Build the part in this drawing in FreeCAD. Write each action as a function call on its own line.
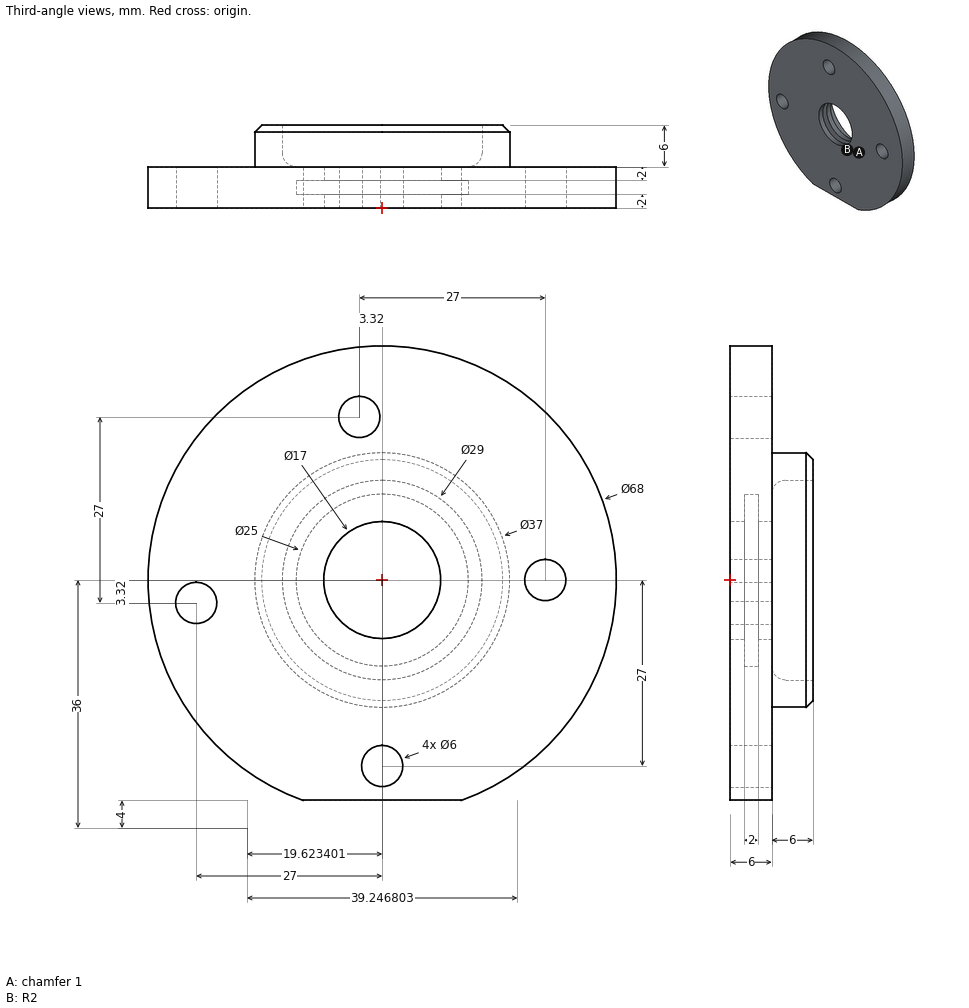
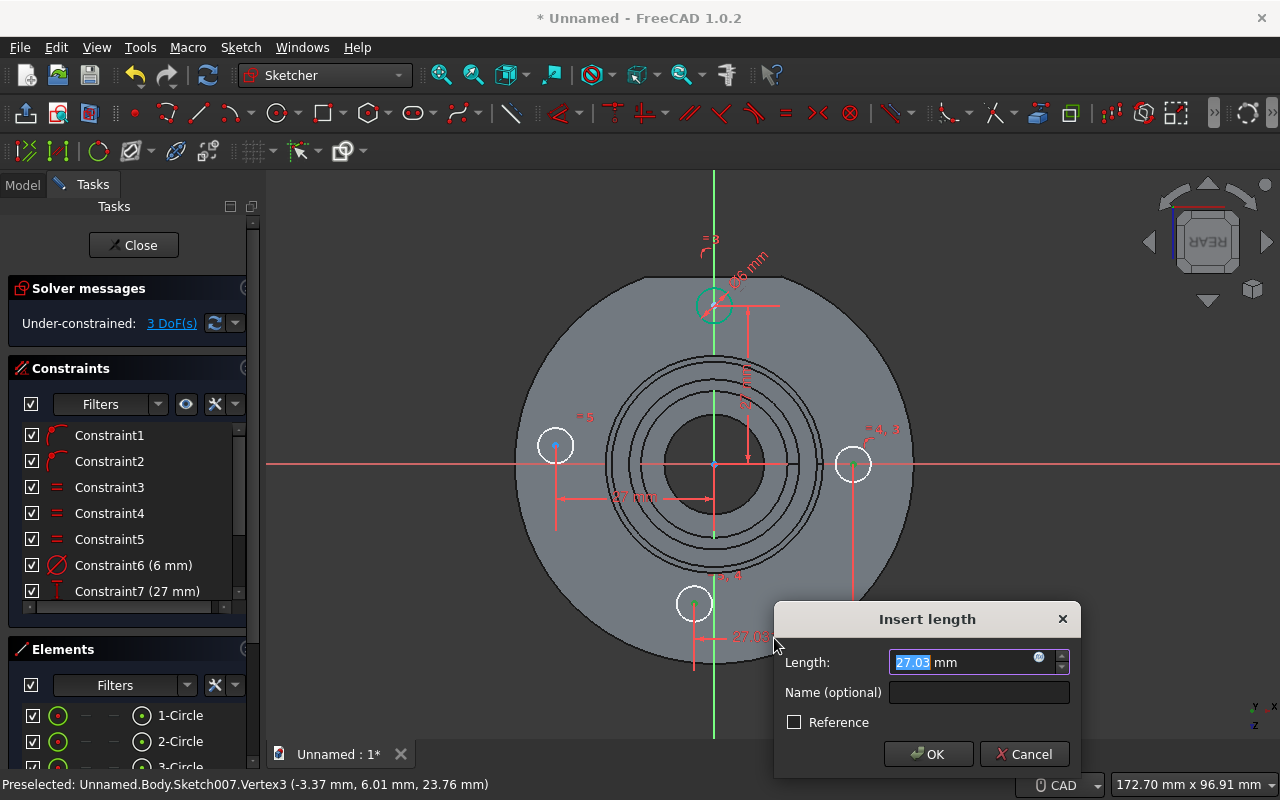
text(27)
key(Return)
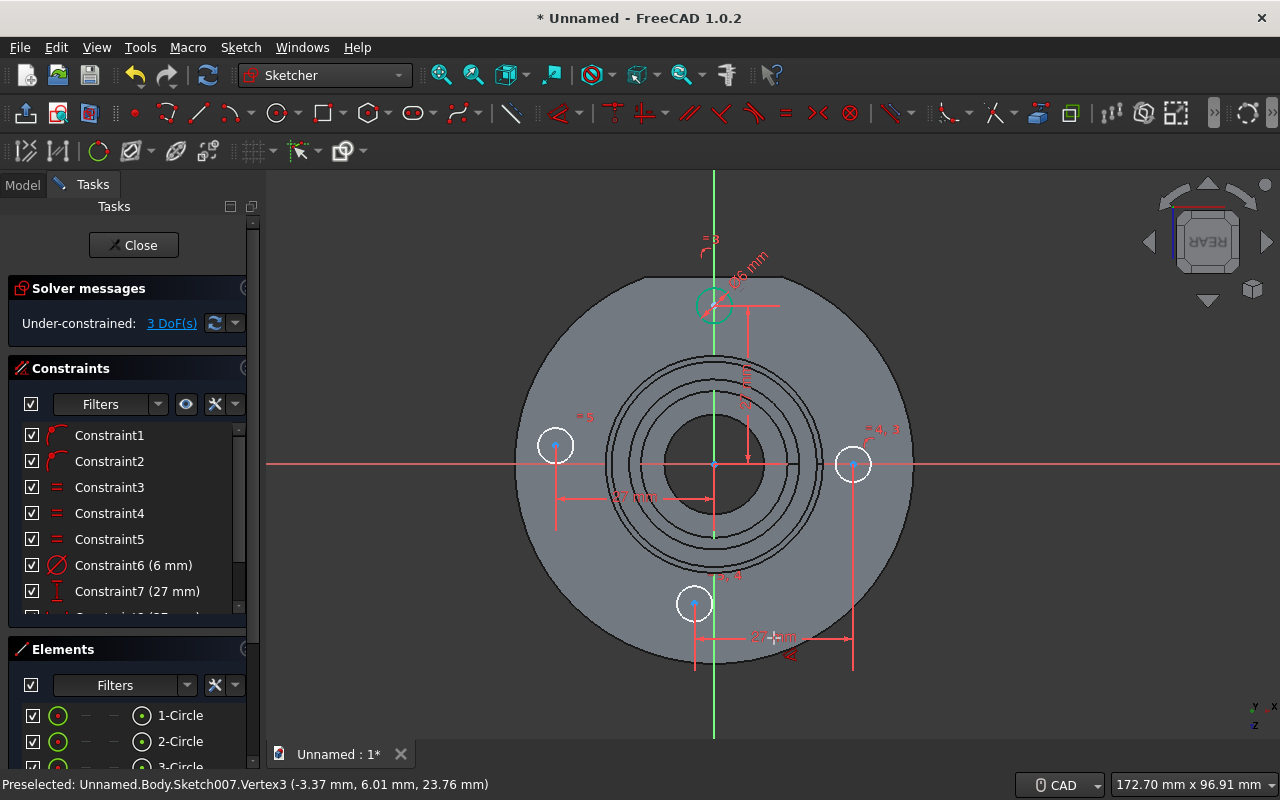
click(695, 604)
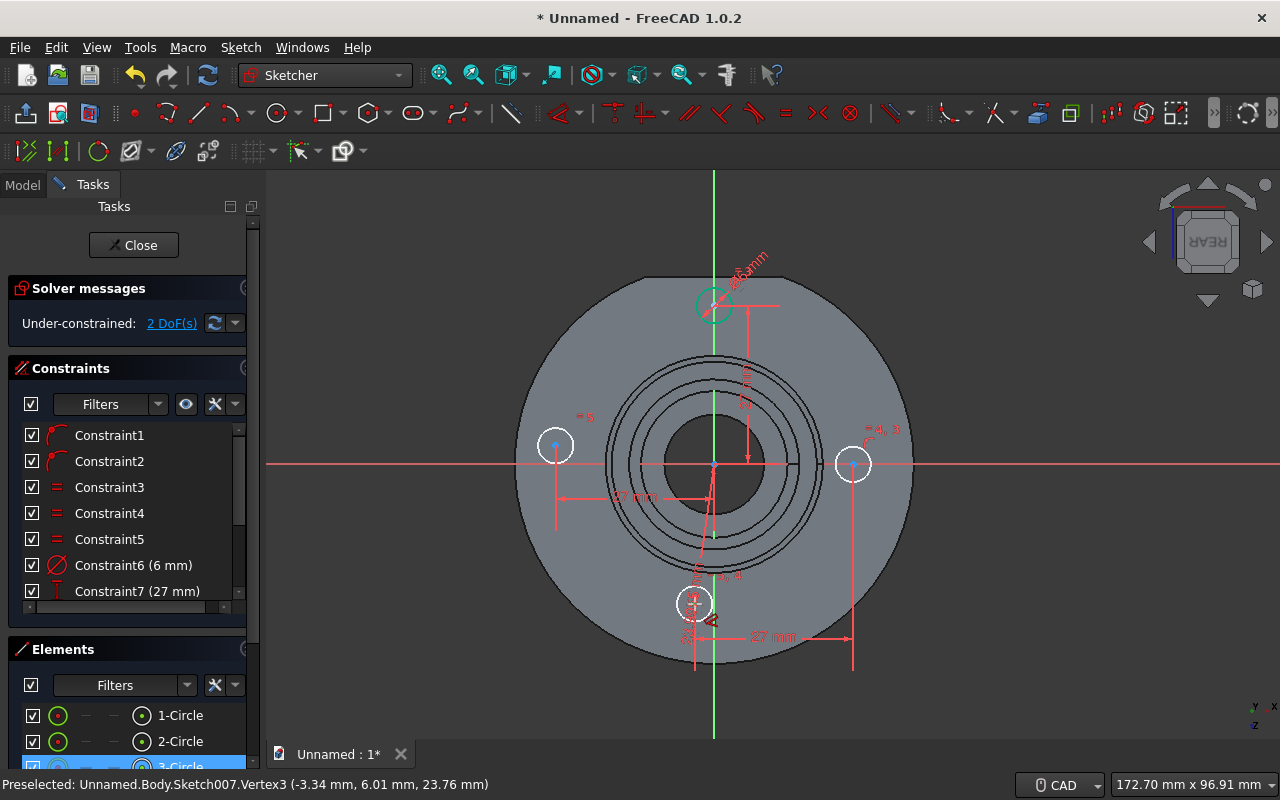
click(556, 446)
click(522, 525)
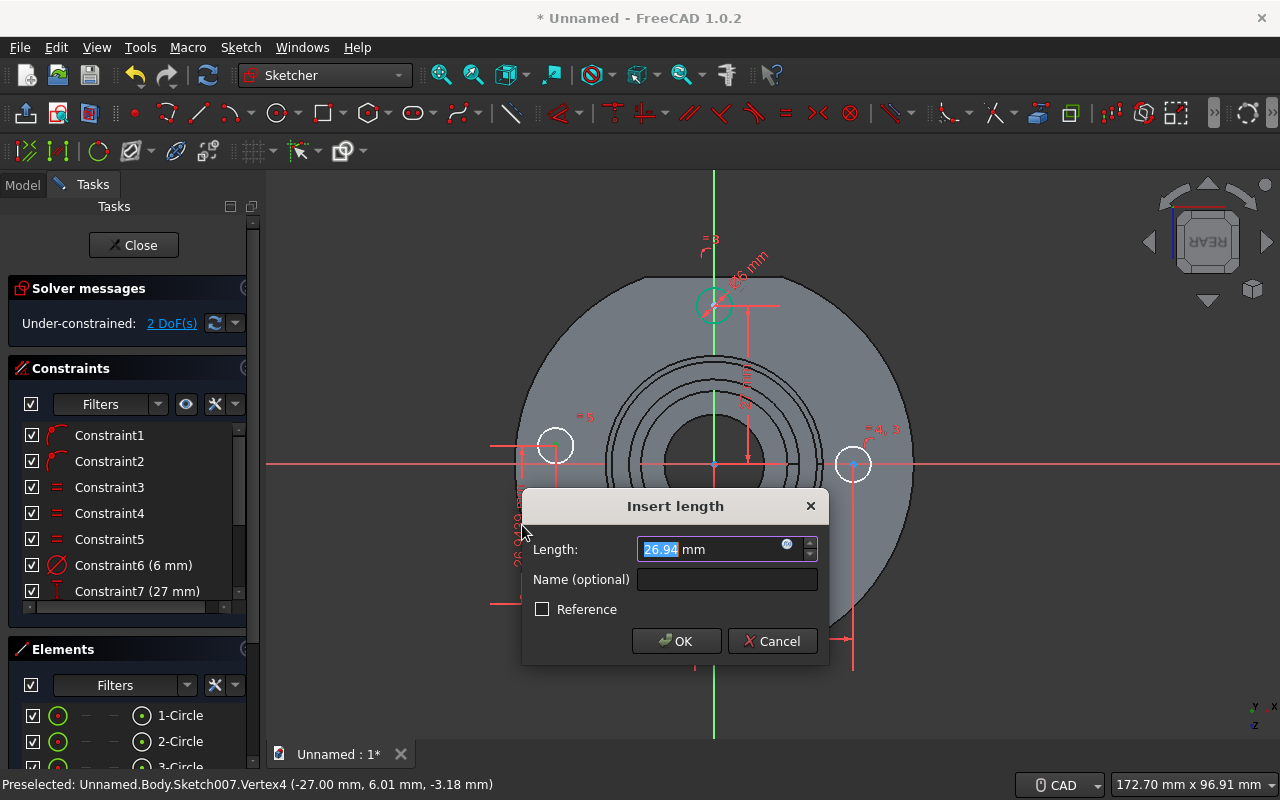
text(27)
key(Return)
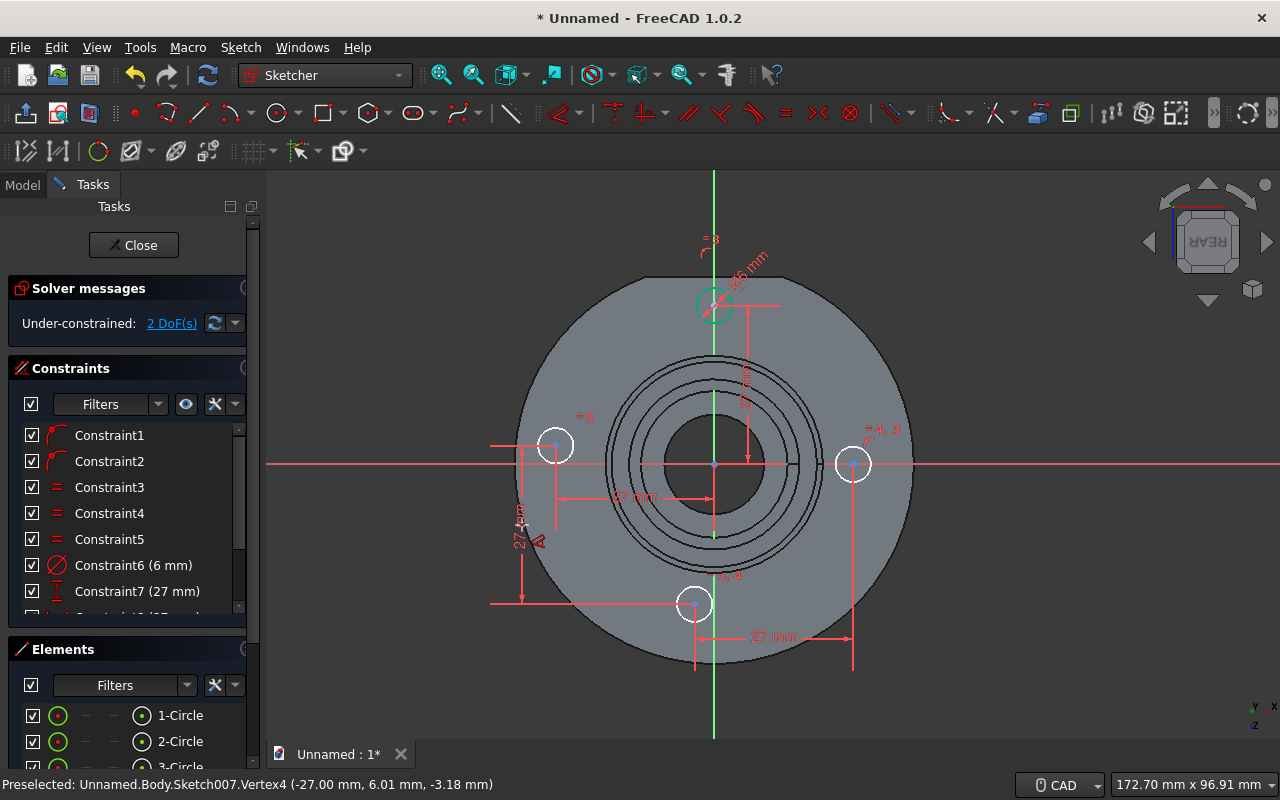
scroll(695, 604, up, 4)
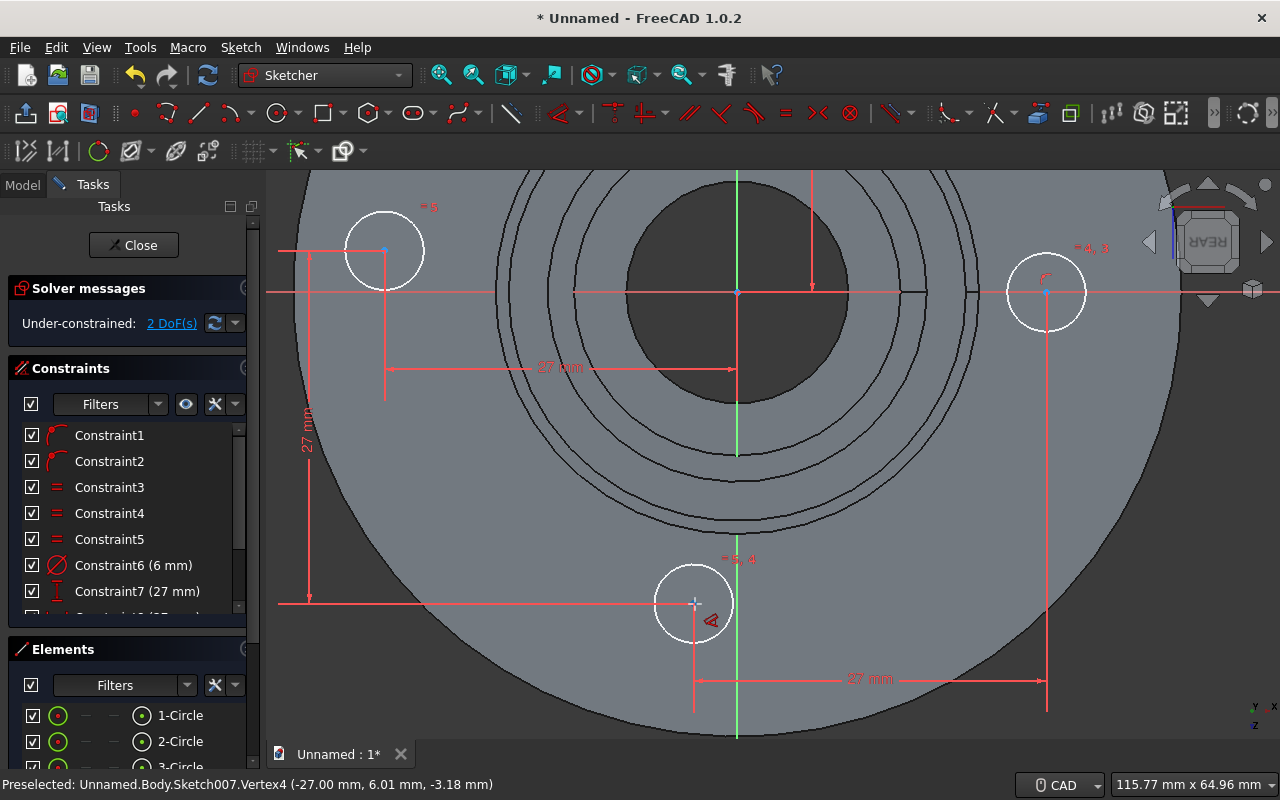
click(694, 604)
click(716, 258)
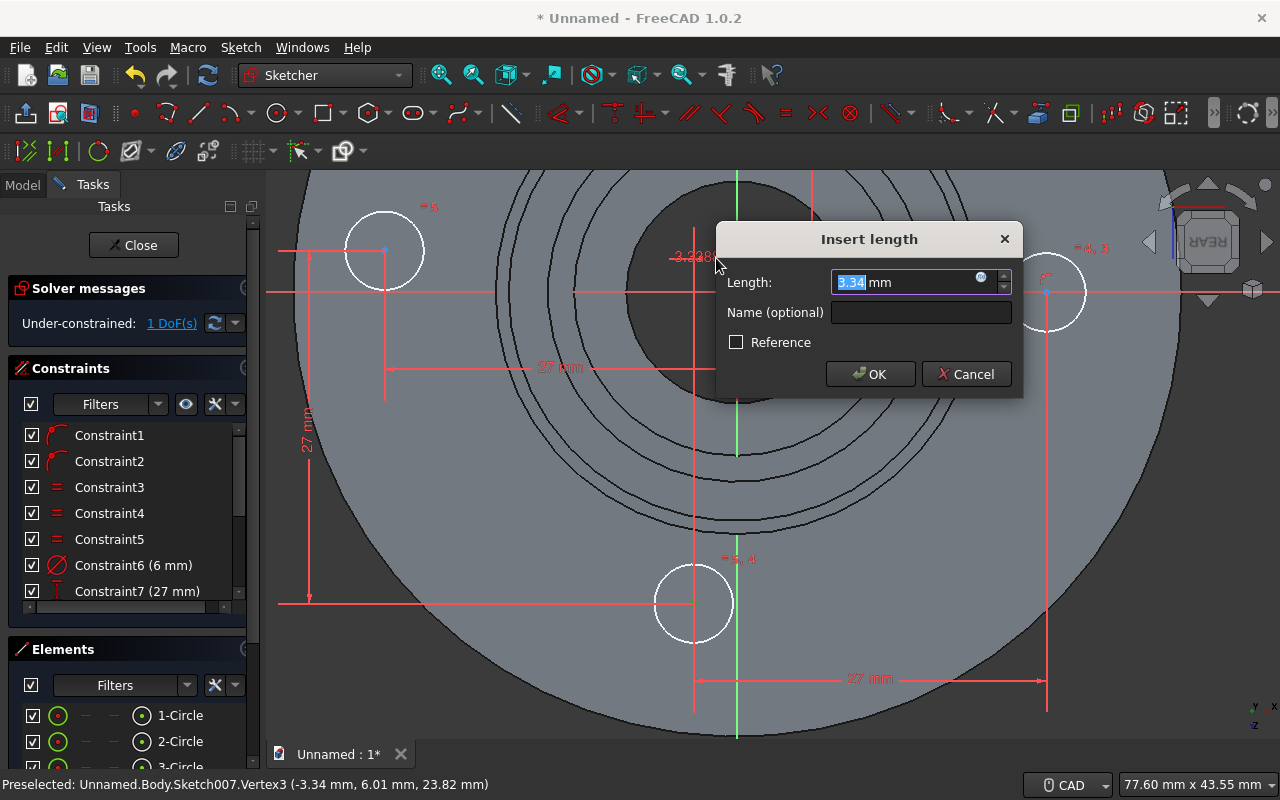
text(3.32)
key(Return)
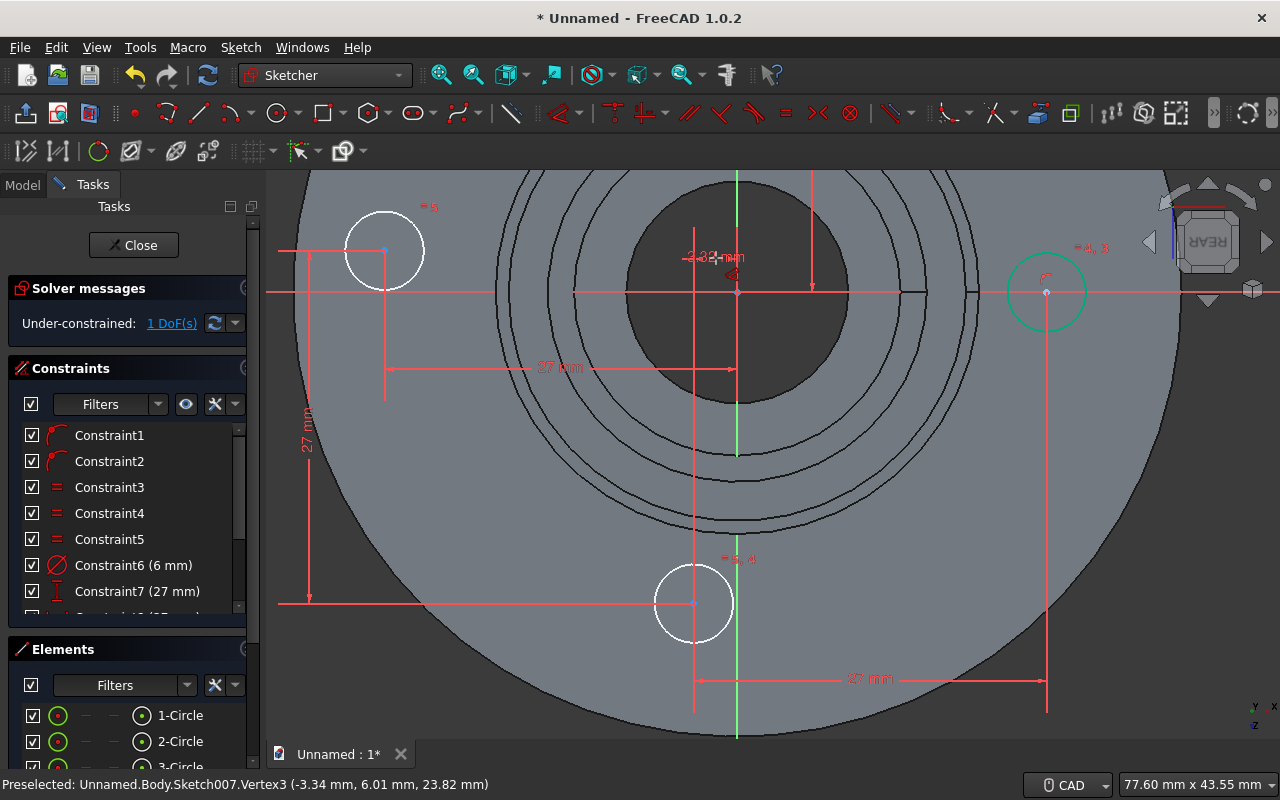
click(385, 251)
click(327, 272)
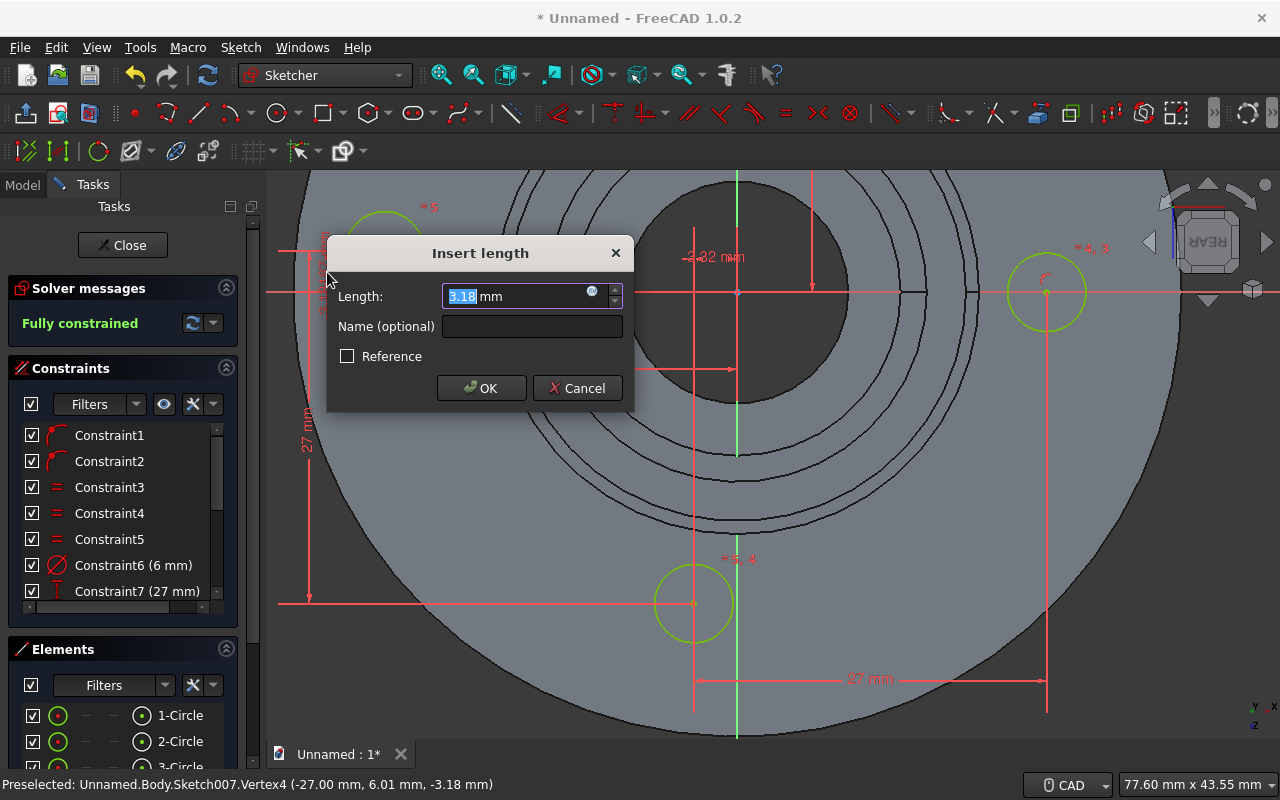
text(3.32)
key(Return)
key(Escape)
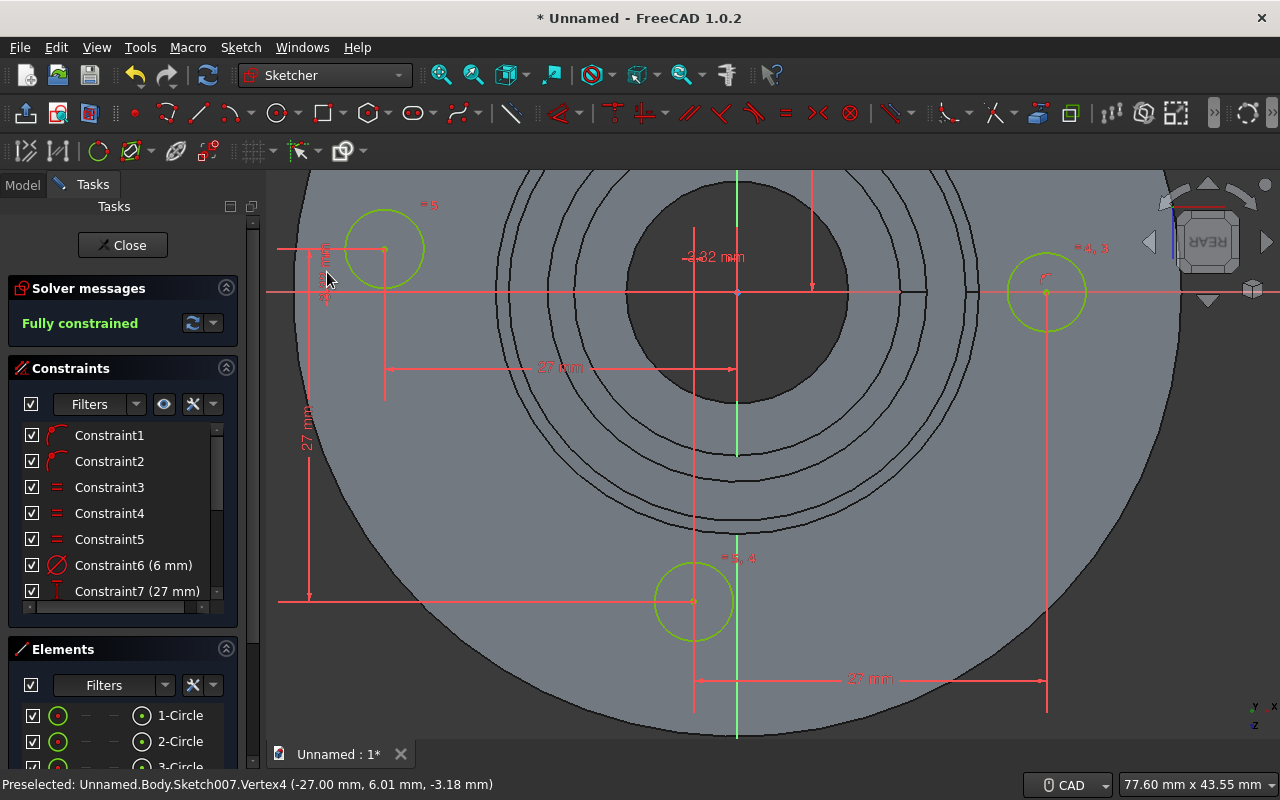
click(123, 245)